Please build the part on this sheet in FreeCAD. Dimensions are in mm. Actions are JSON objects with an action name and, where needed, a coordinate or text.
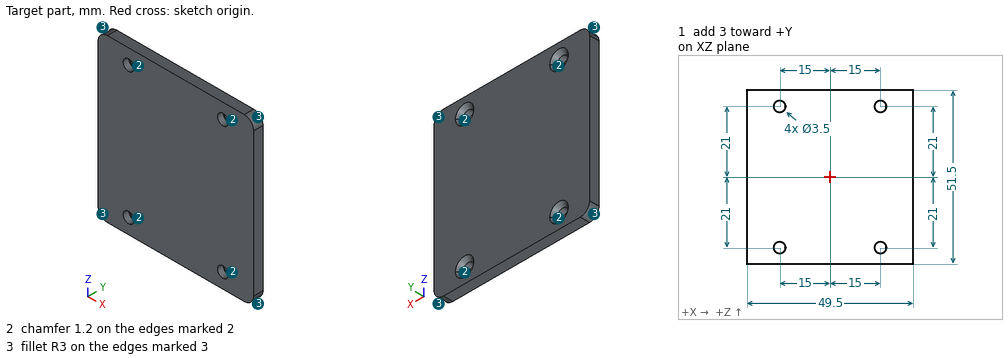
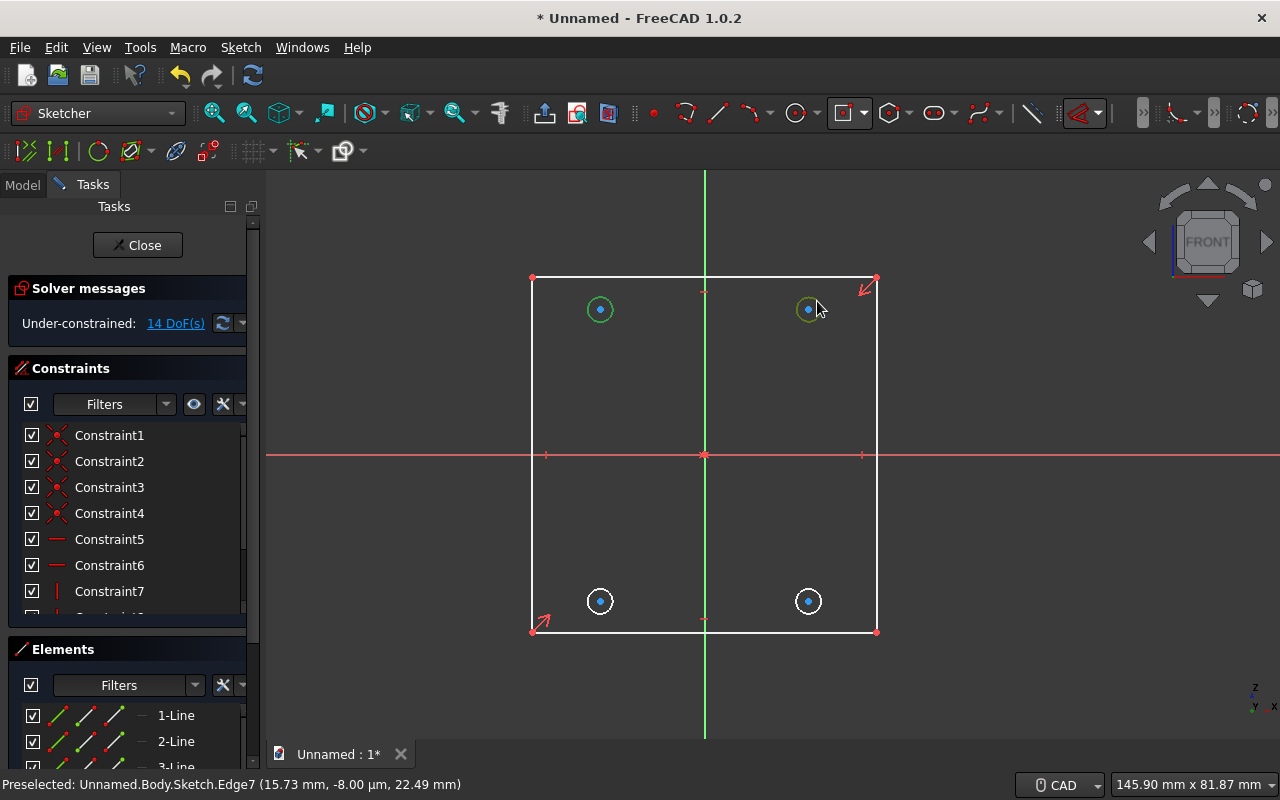
{"action": "left_click", "coordinate": [609, 593]}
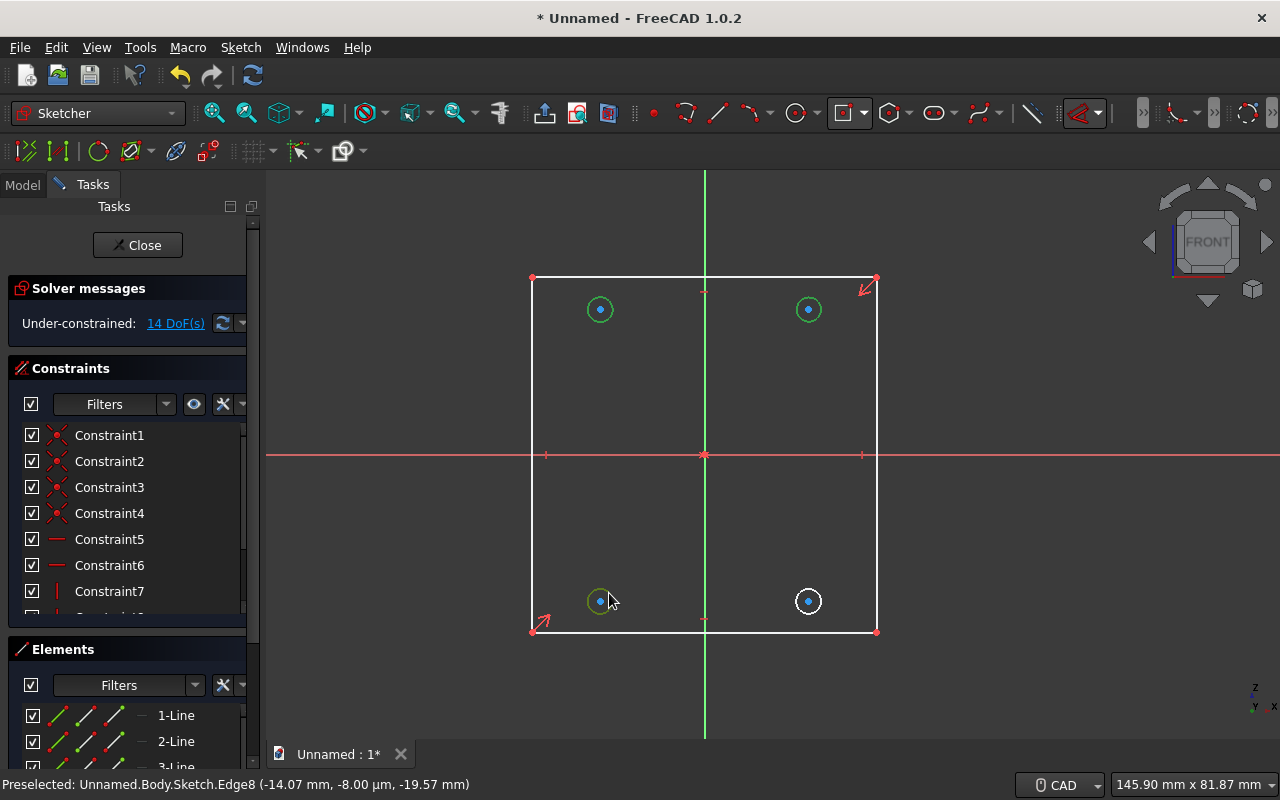
{"action": "left_click", "coordinate": [817, 593]}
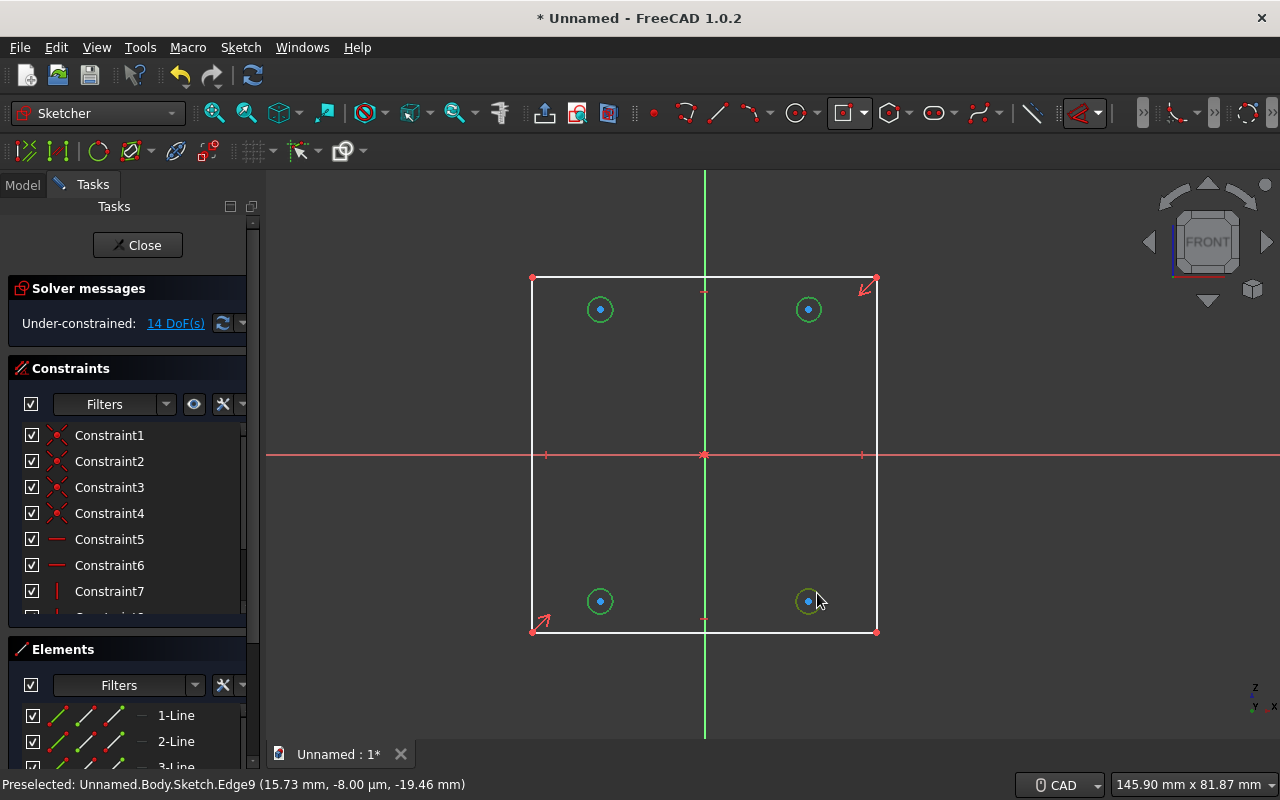
{"action": "key", "text": "e"}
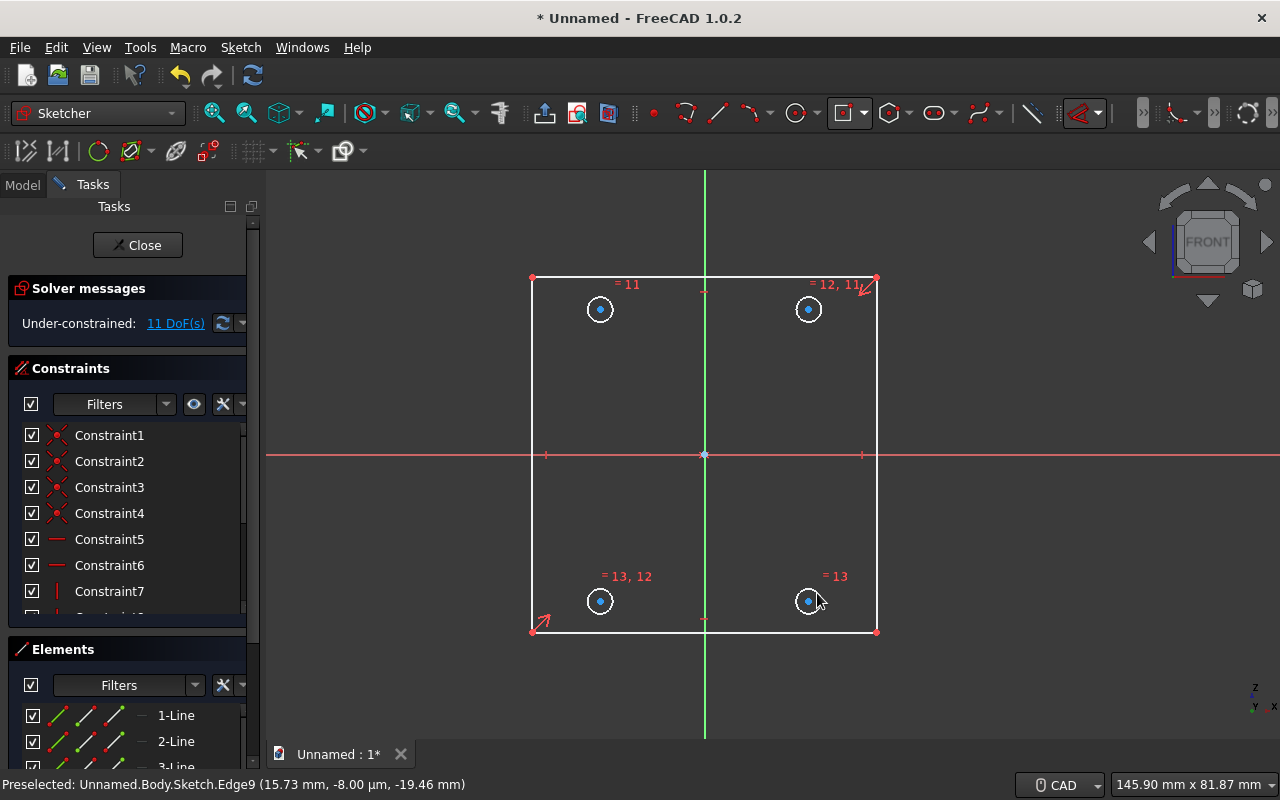
{"action": "left_click", "coordinate": [1078, 114]}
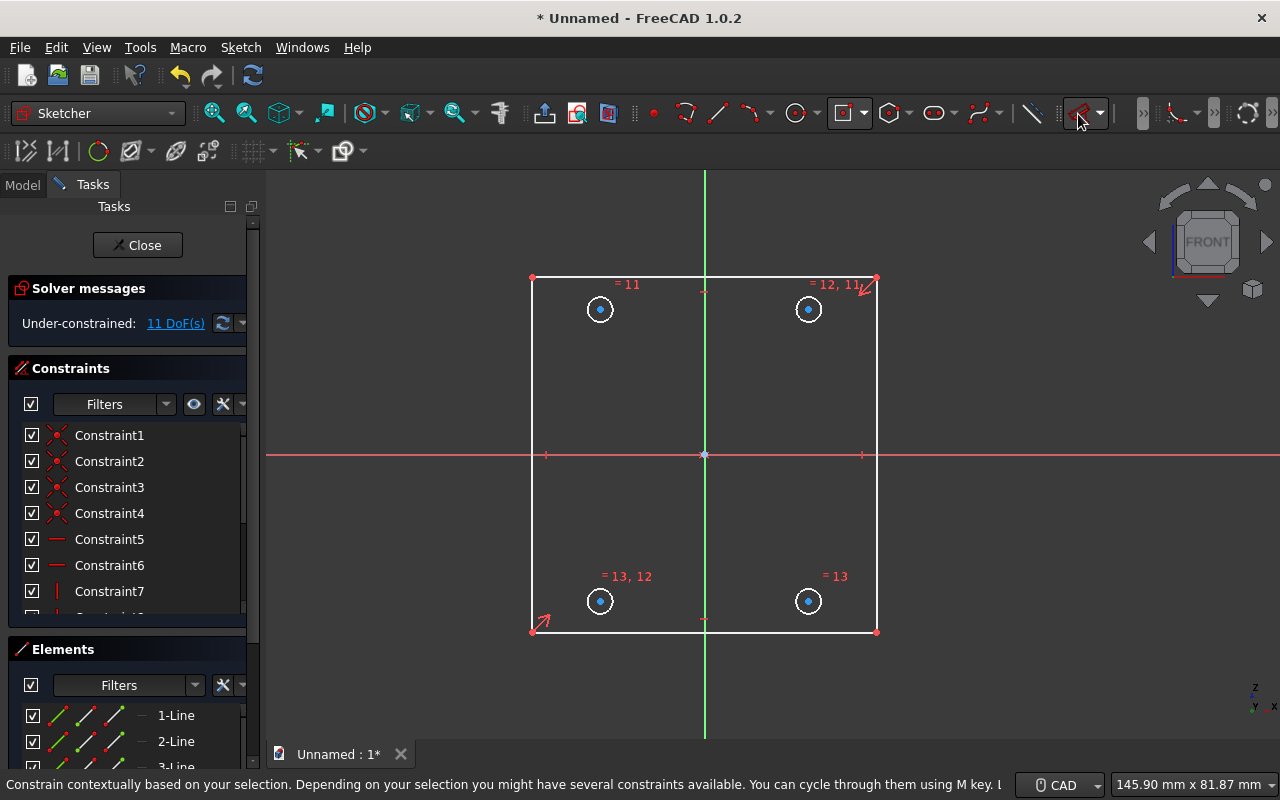
{"action": "scroll", "coordinate": [609, 301], "scroll_direction": "up", "scroll_amount": 3}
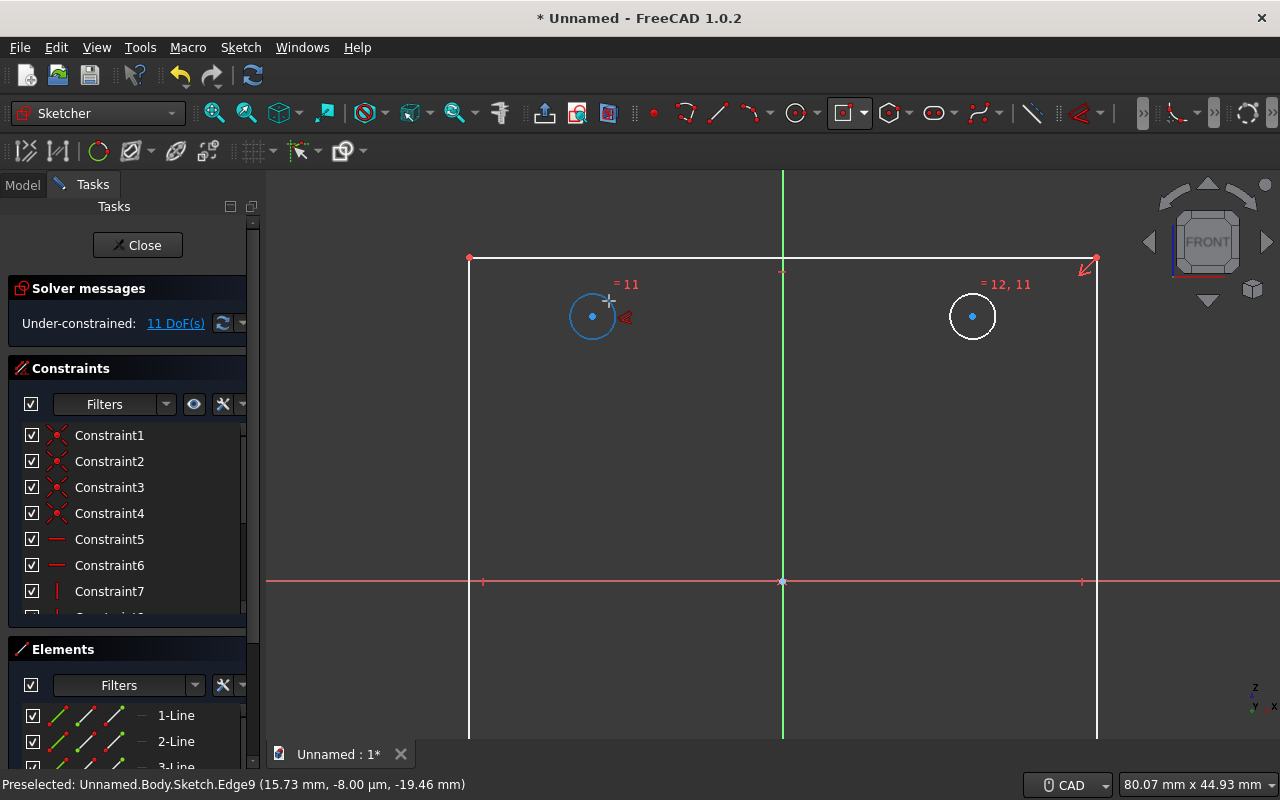
{"action": "left_click", "coordinate": [609, 301]}
{"action": "left_click", "coordinate": [632, 279]}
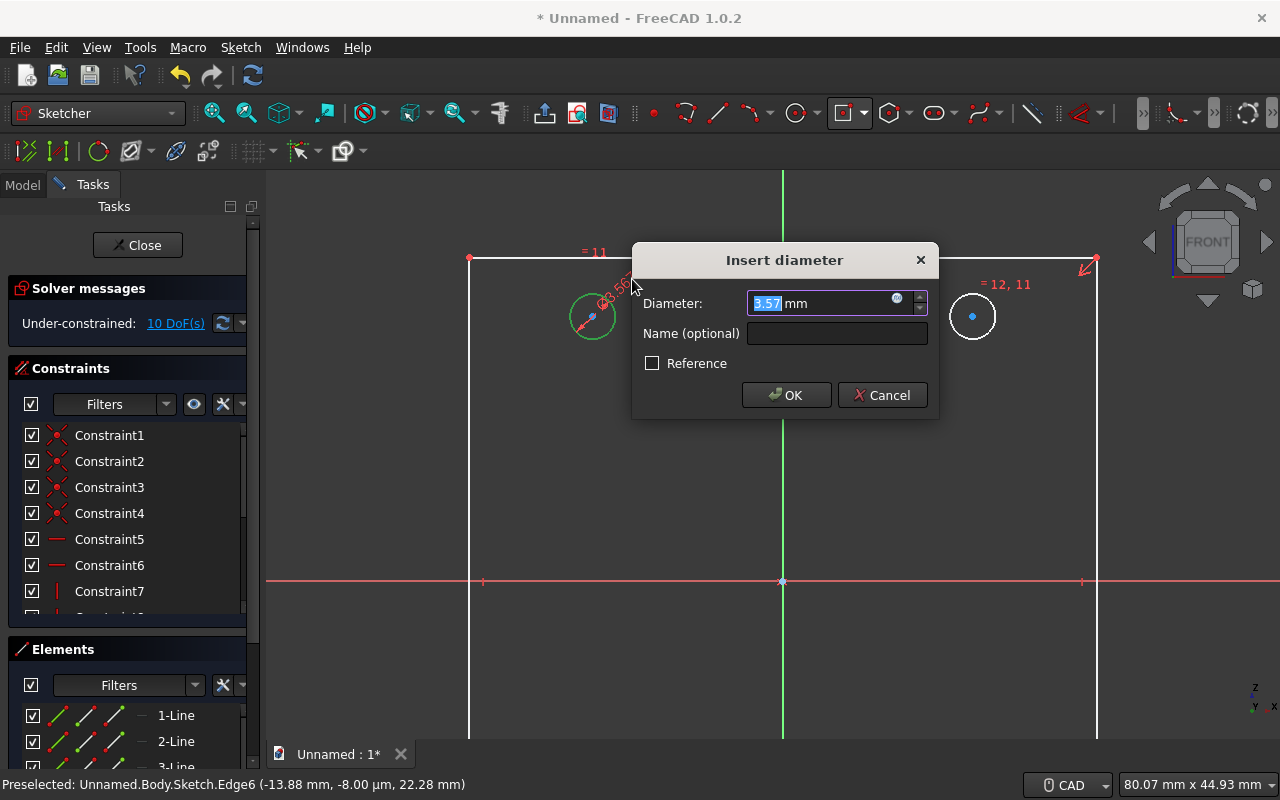
{"action": "type", "text": "3.5"}
{"action": "key", "text": "Return"}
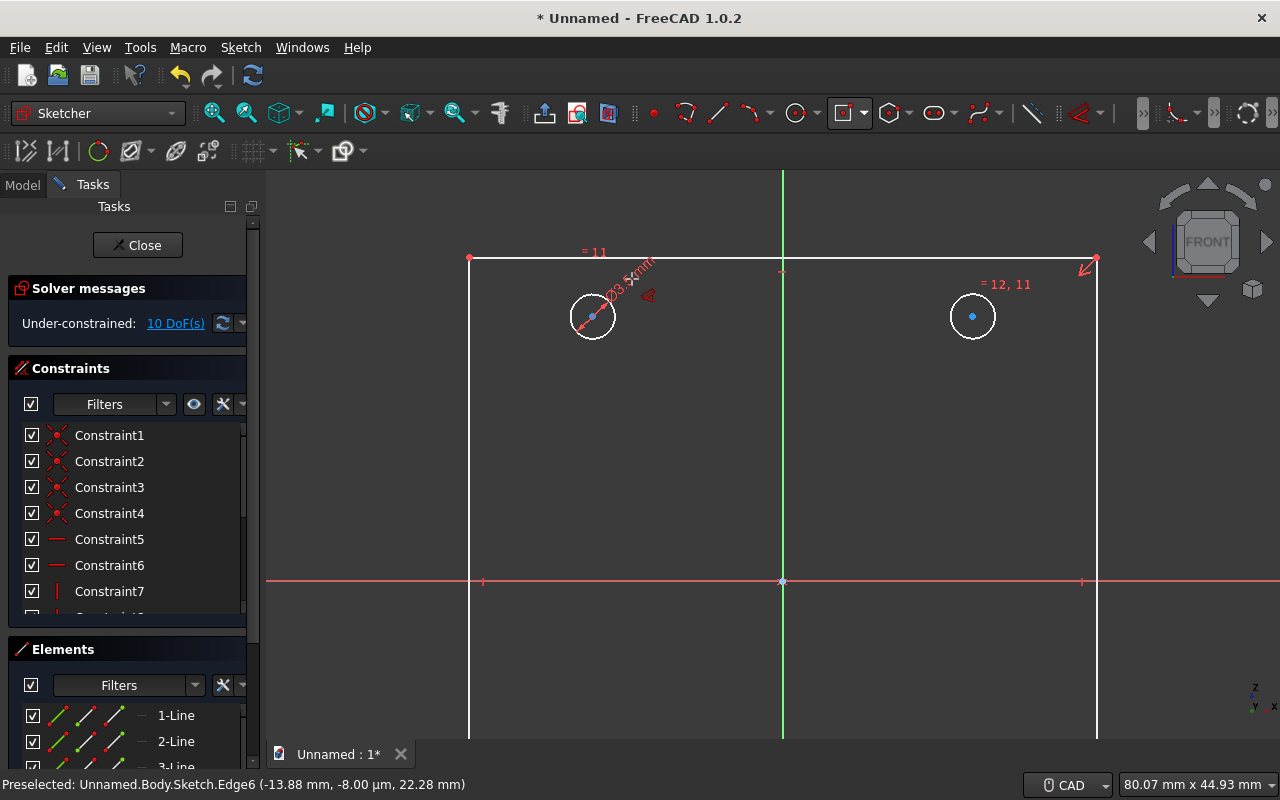
{"action": "left_click", "coordinate": [593, 317]}
{"action": "left_click", "coordinate": [732, 283]}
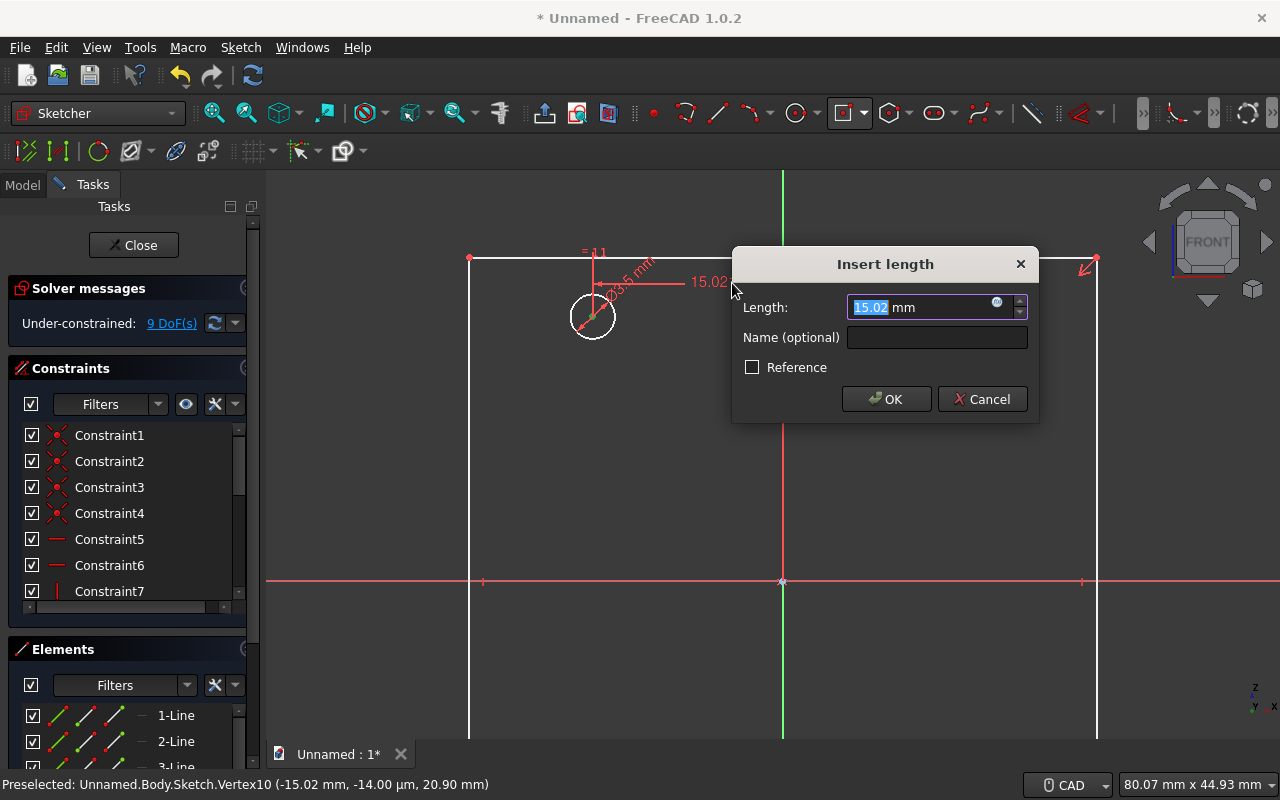
{"action": "type", "text": "15"}
{"action": "key", "text": "Return"}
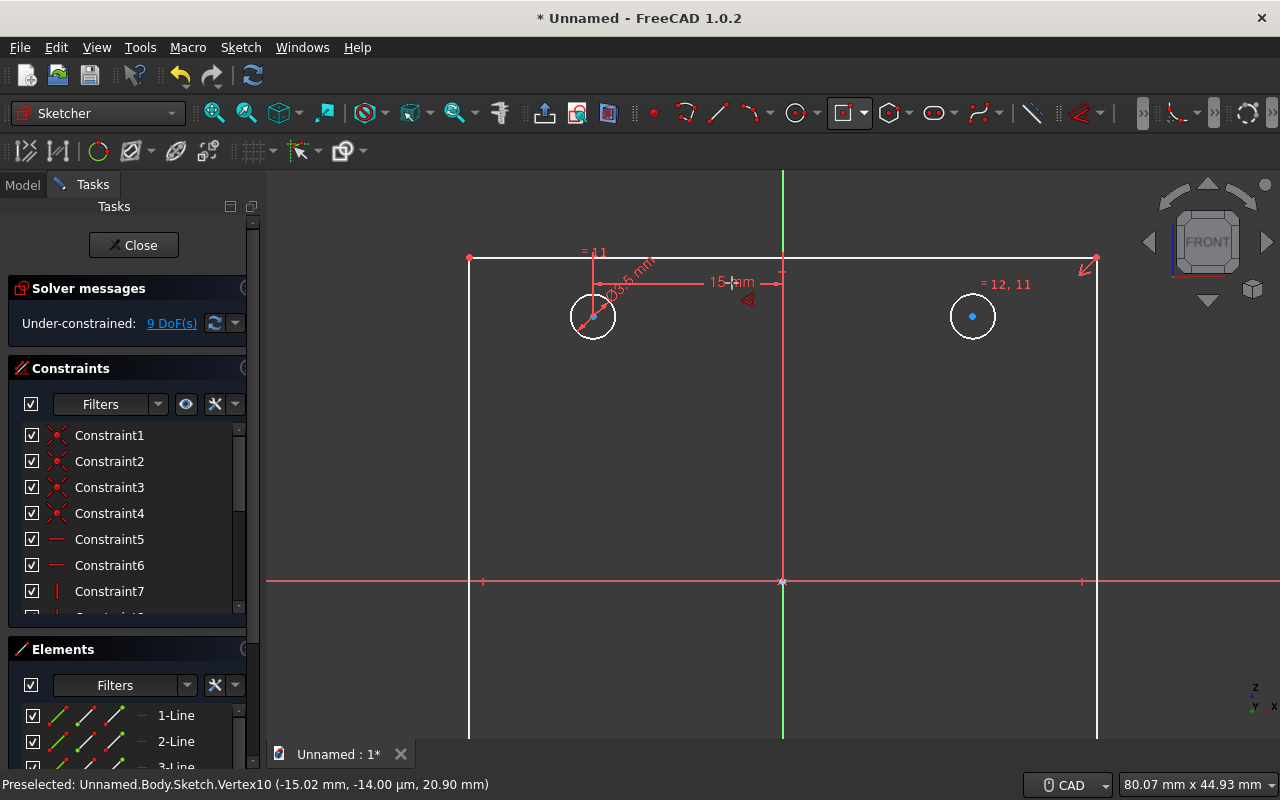
{"action": "left_click", "coordinate": [593, 317]}
{"action": "left_click", "coordinate": [559, 449]}